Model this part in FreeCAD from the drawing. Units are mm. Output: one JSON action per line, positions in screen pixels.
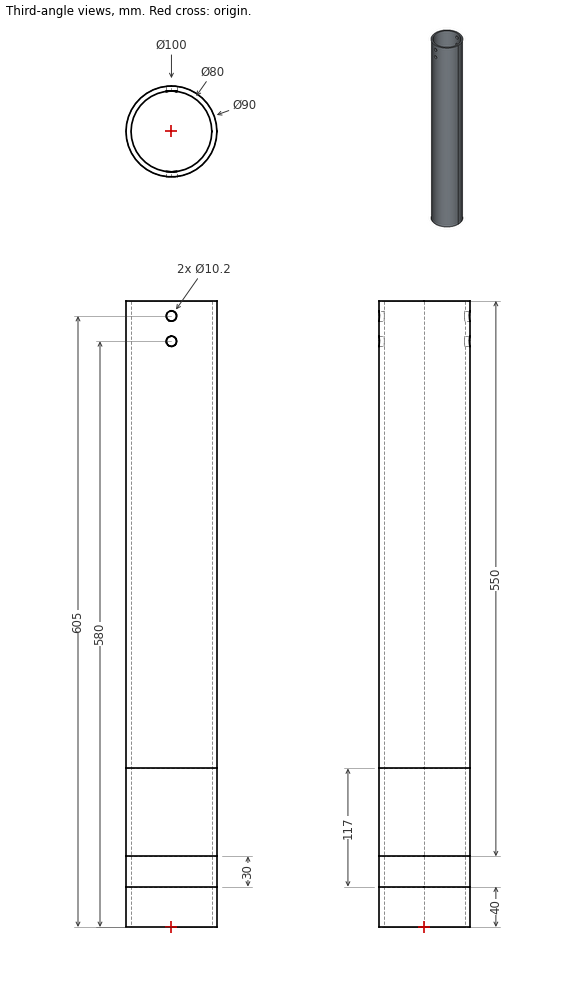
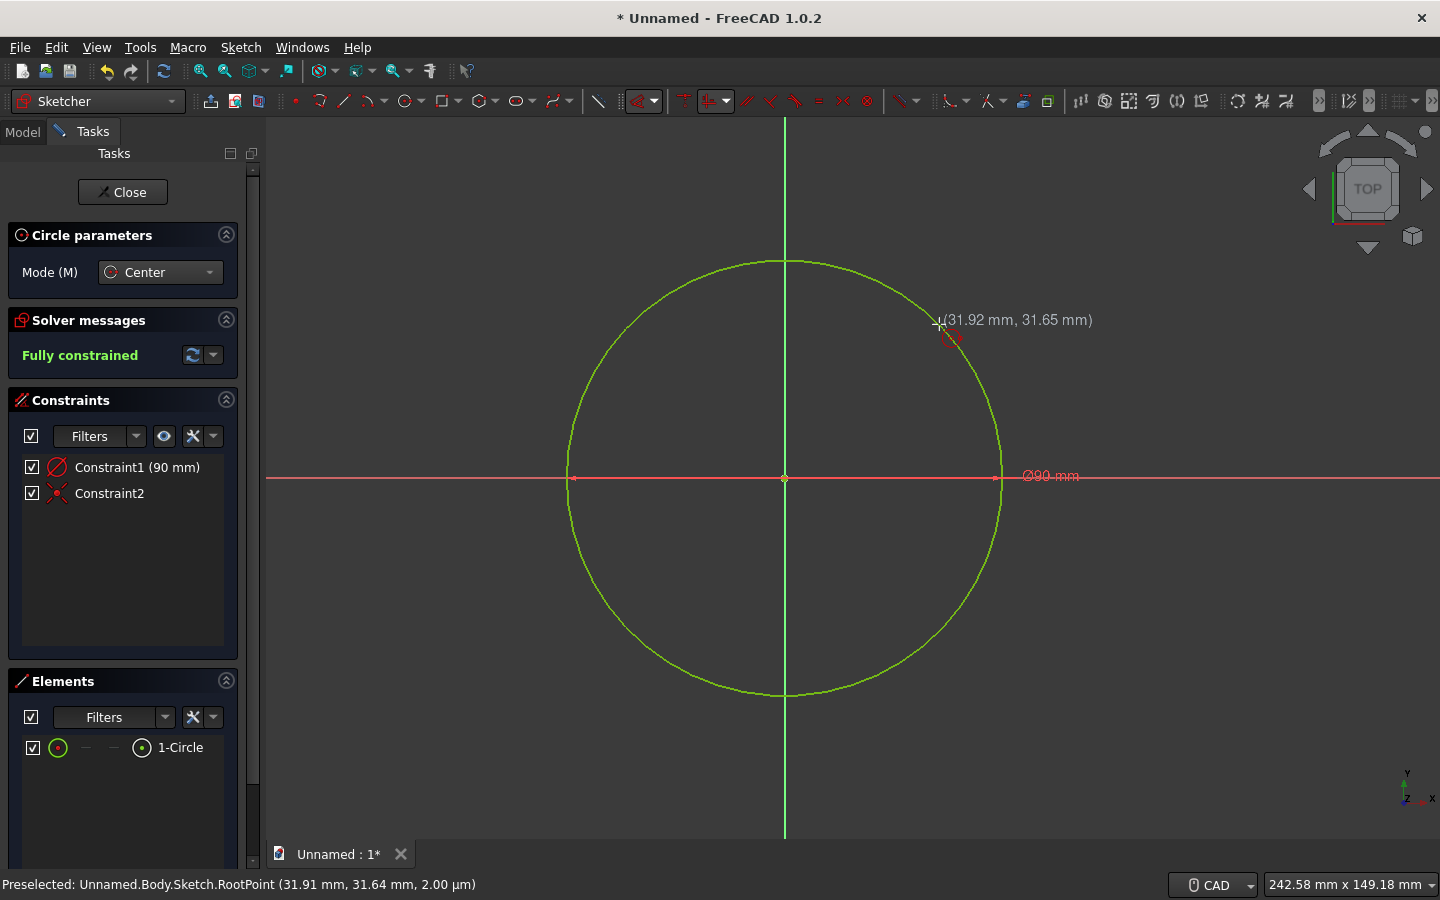
{"action": "left_click", "coordinate": [785, 478]}
{"action": "mouse_move", "coordinate": [921, 341]}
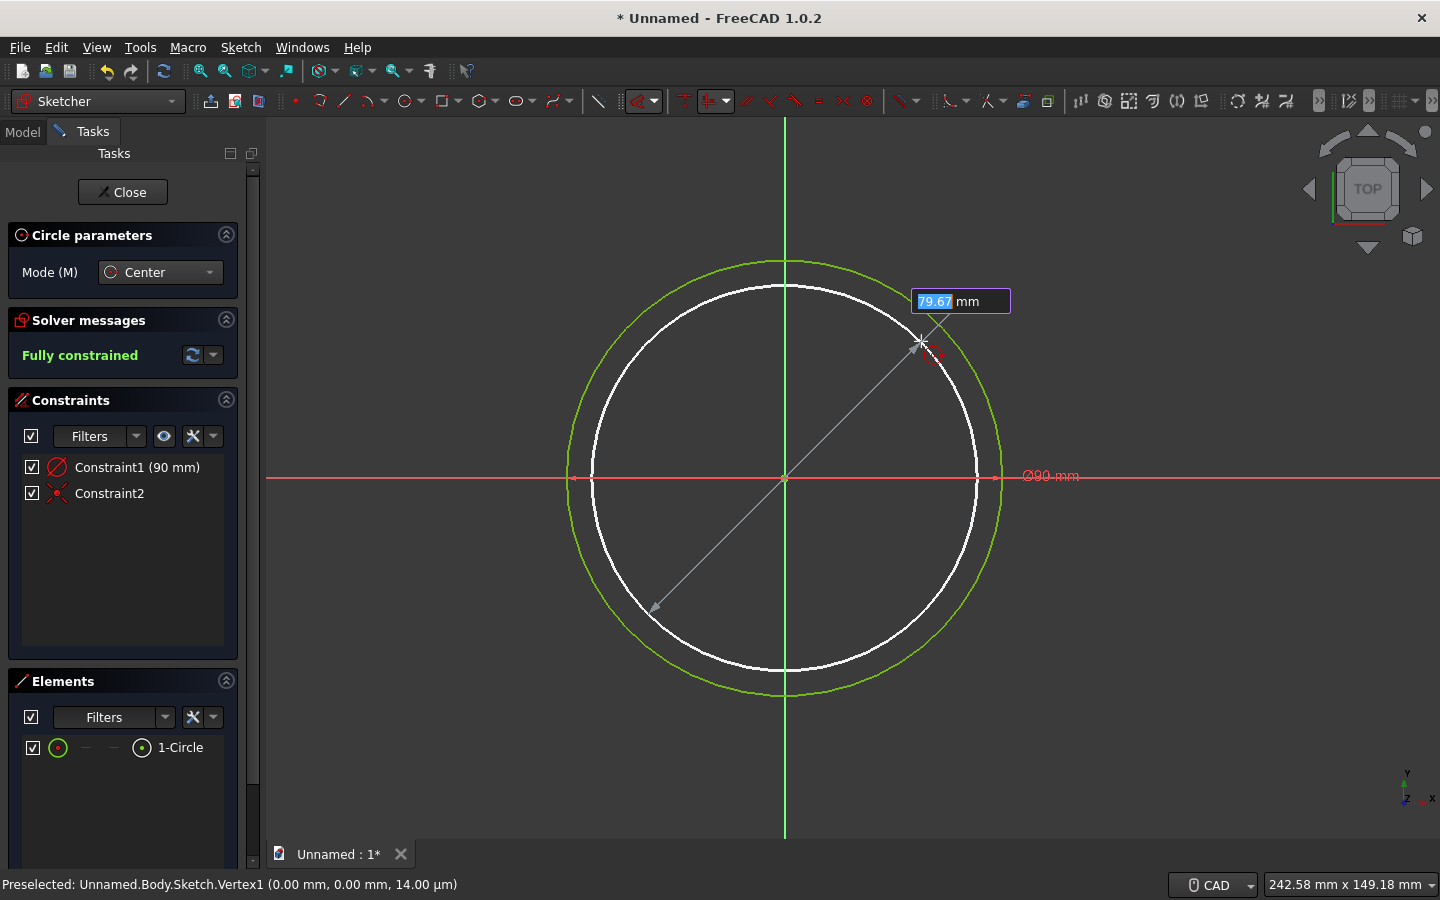
{"action": "type", "text": "80"}
{"action": "key", "text": "Return"}
{"action": "key", "text": "Escape"}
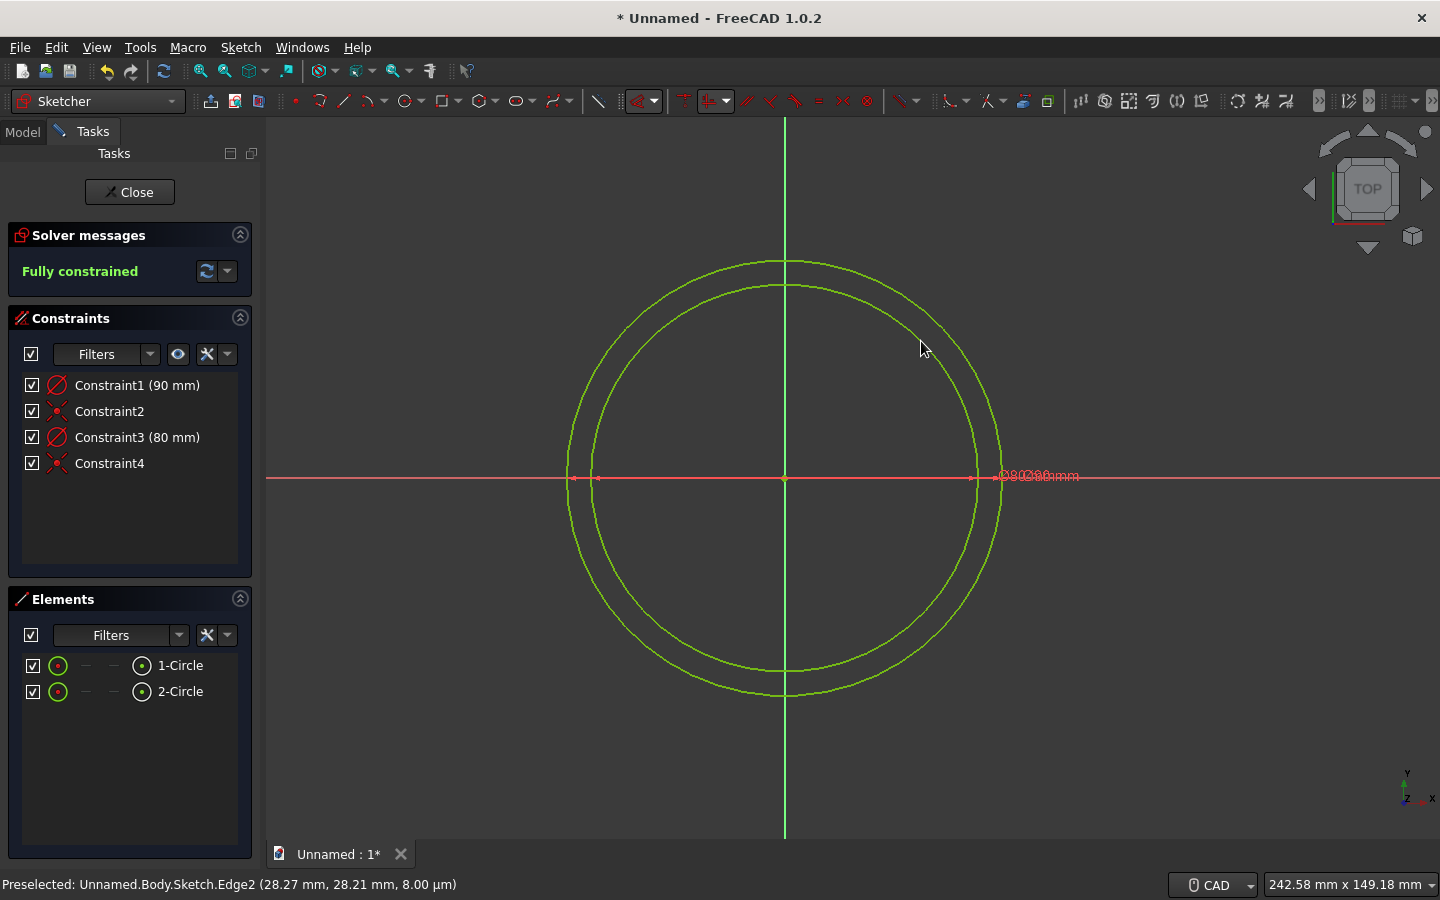
{"action": "left_click", "coordinate": [130, 192]}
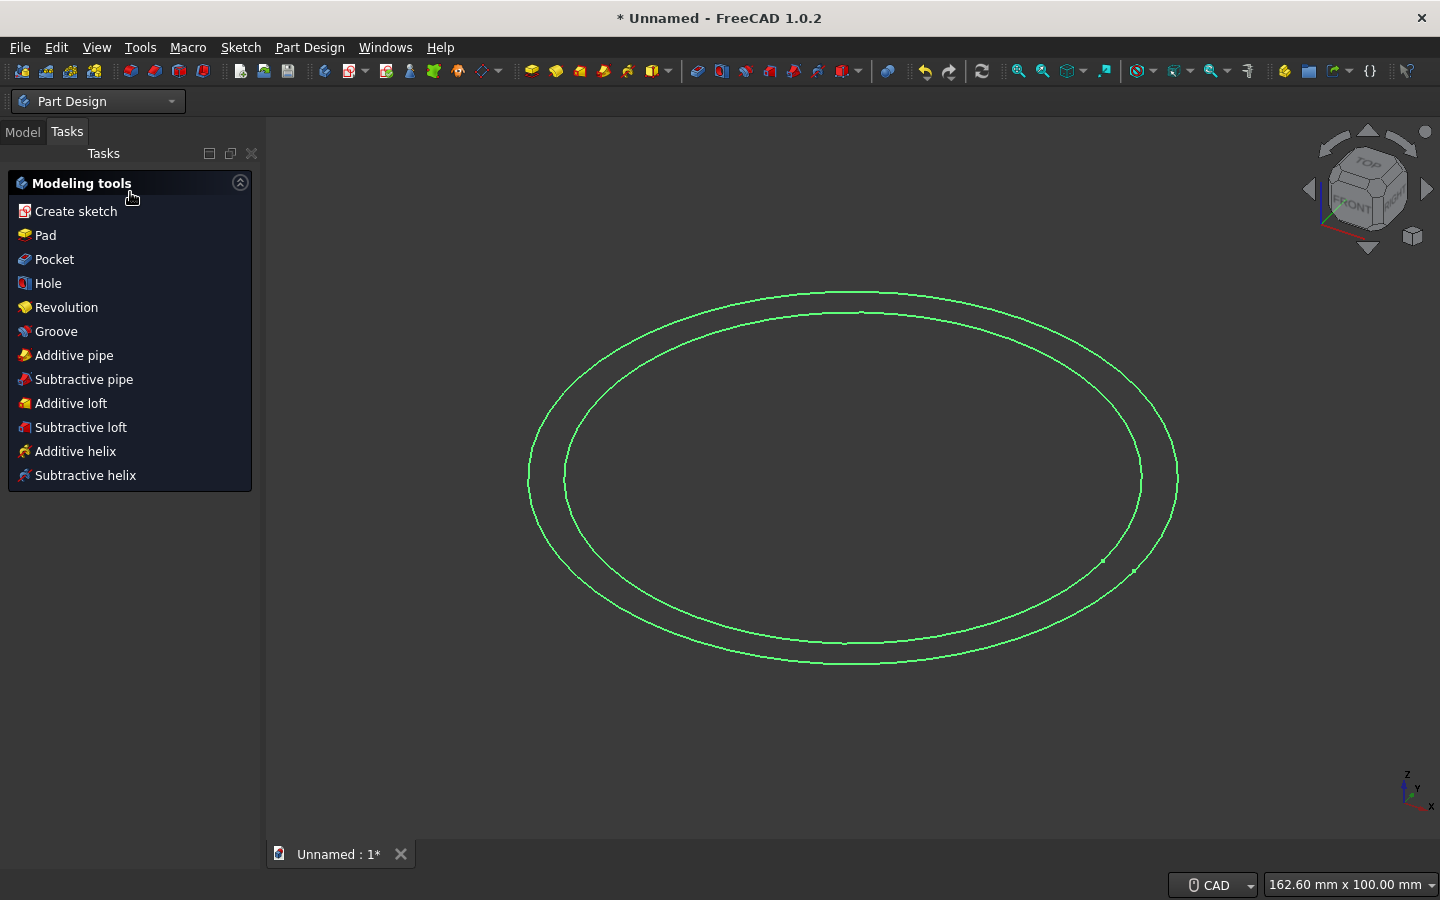
{"action": "left_click", "coordinate": [532, 72]}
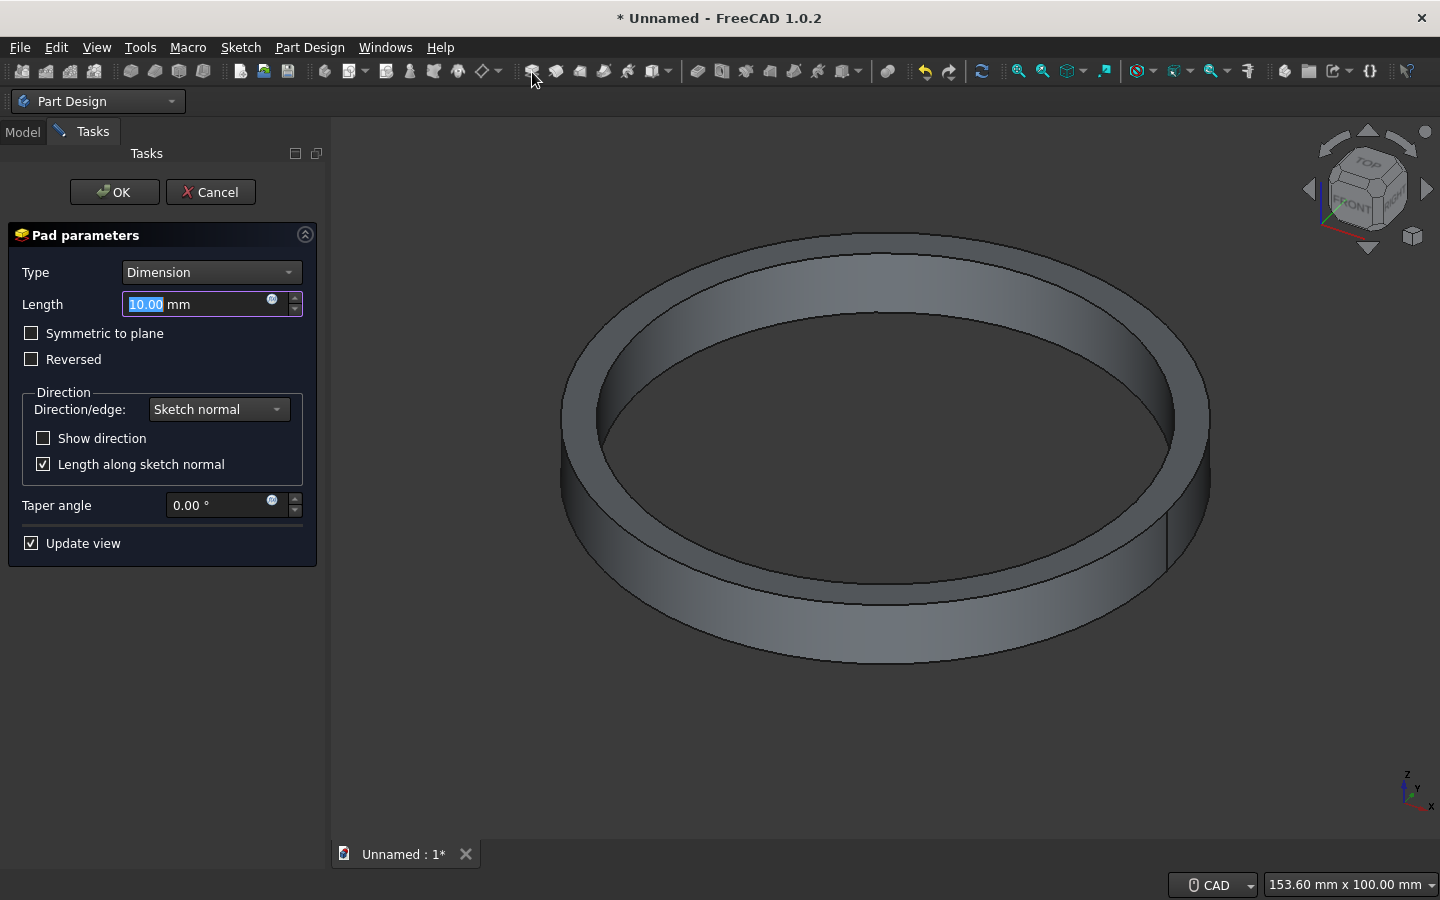
{"action": "type", "text": "40"}
{"action": "key", "text": "Tab"}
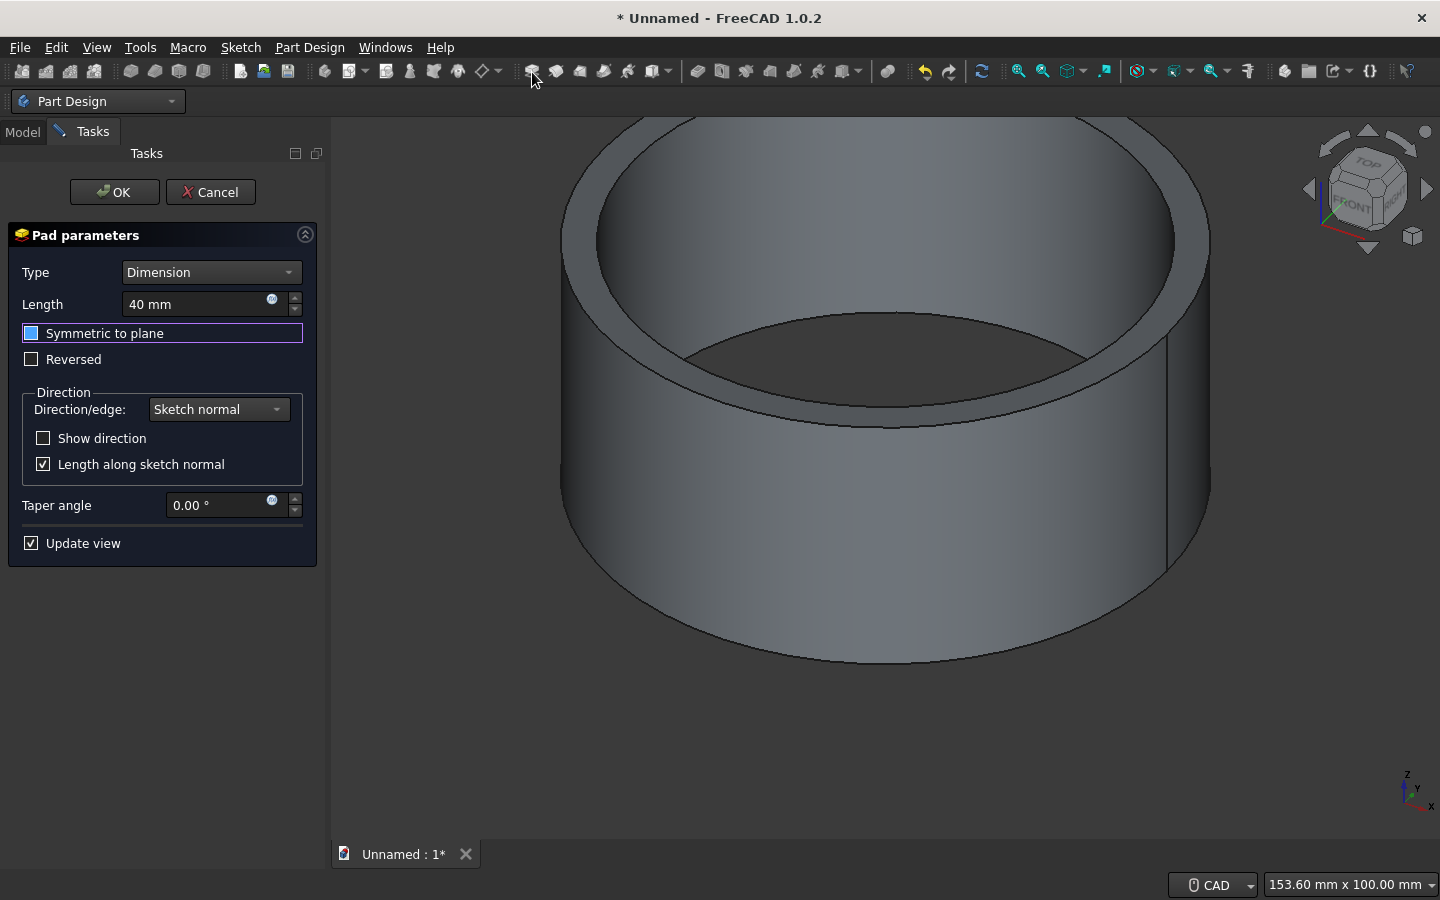
{"action": "left_click", "coordinate": [115, 192]}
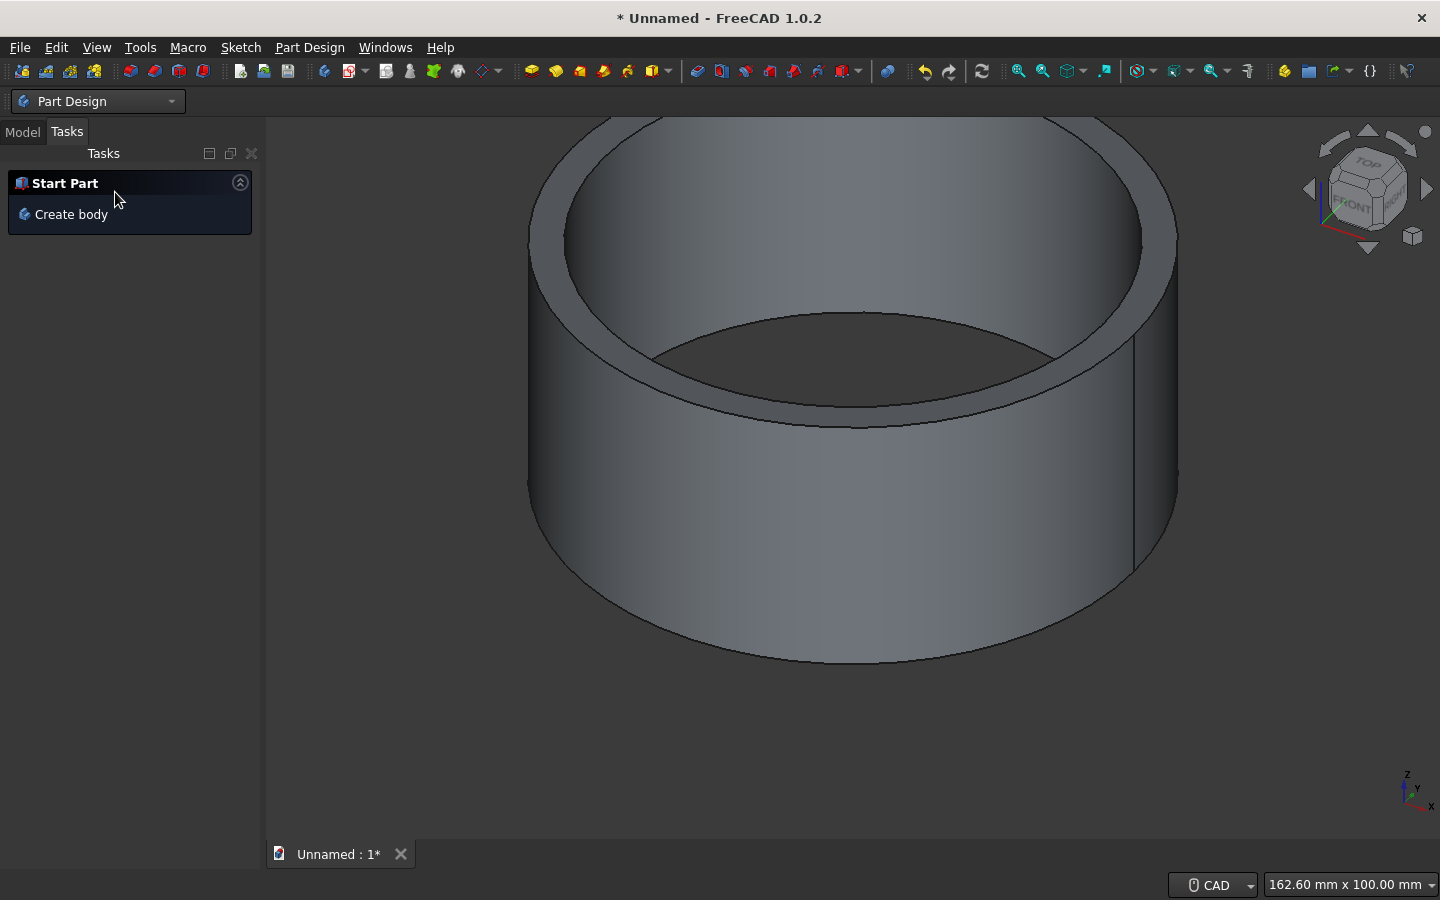
{"action": "key", "text": "v f"}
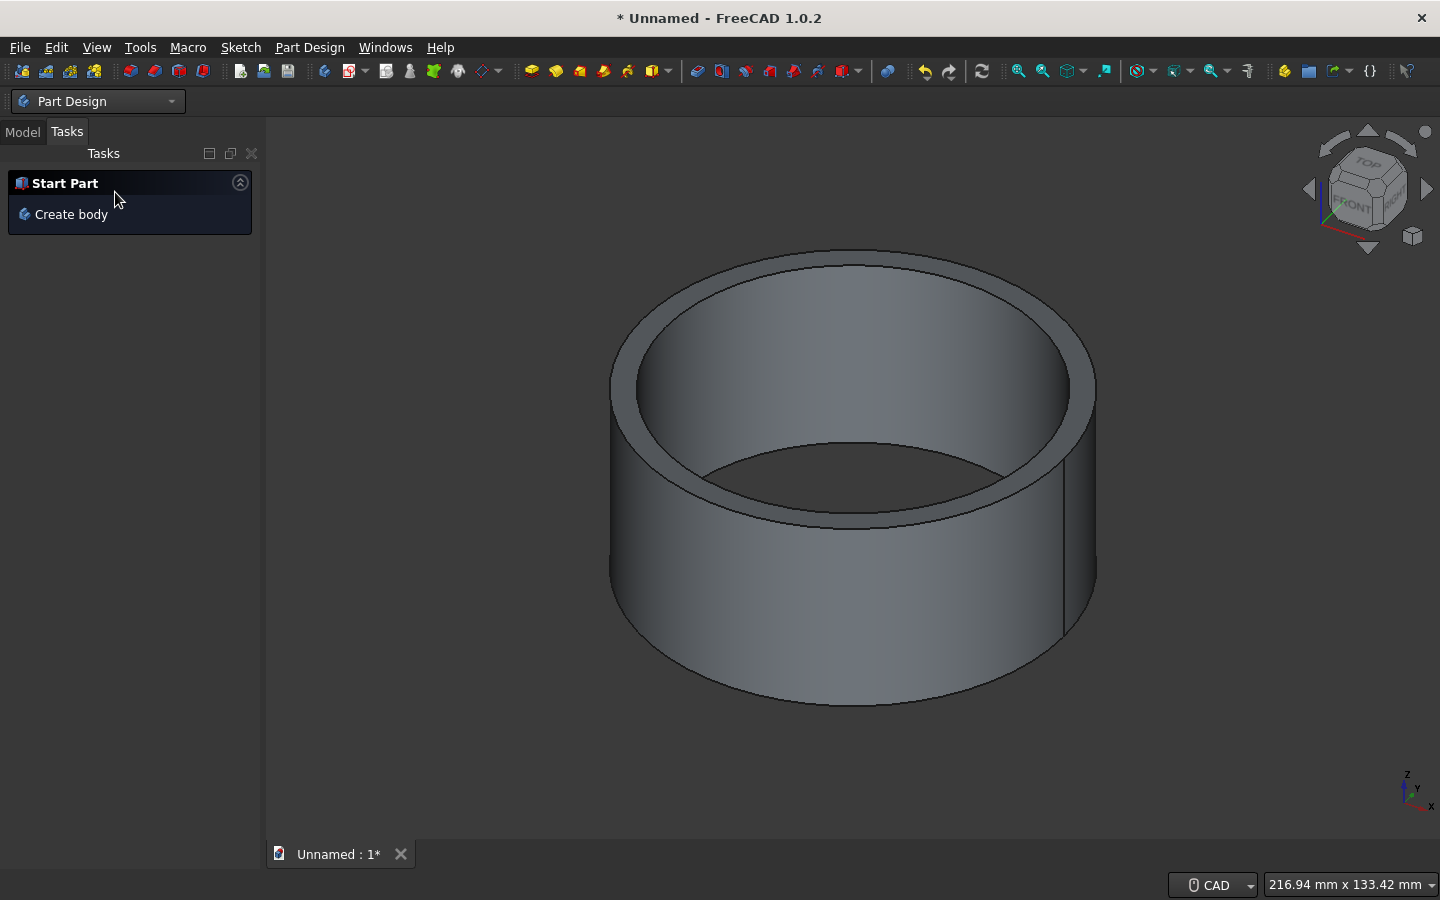
{"action": "left_click", "coordinate": [1069, 414]}